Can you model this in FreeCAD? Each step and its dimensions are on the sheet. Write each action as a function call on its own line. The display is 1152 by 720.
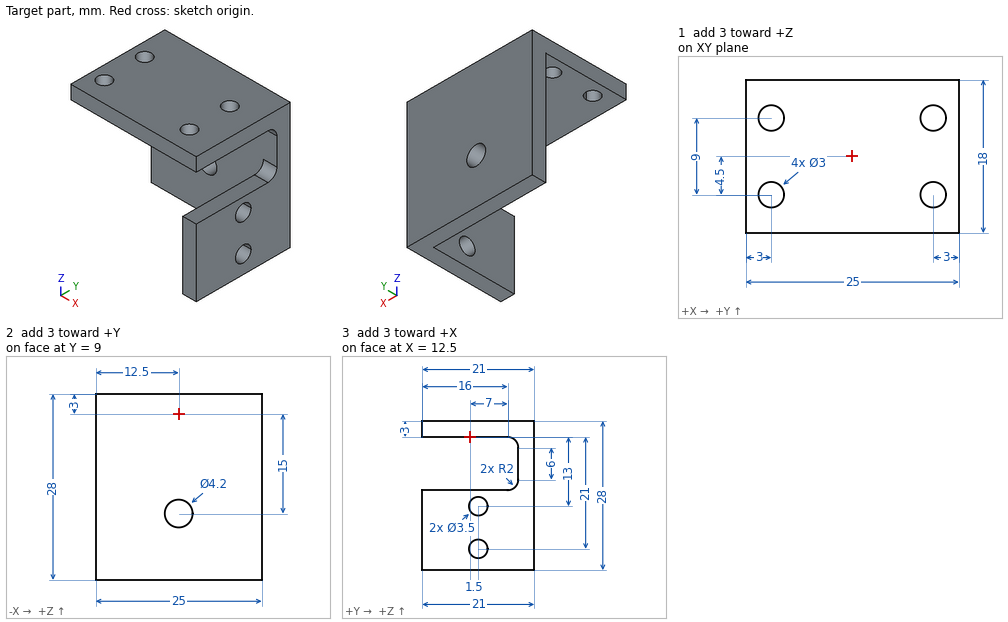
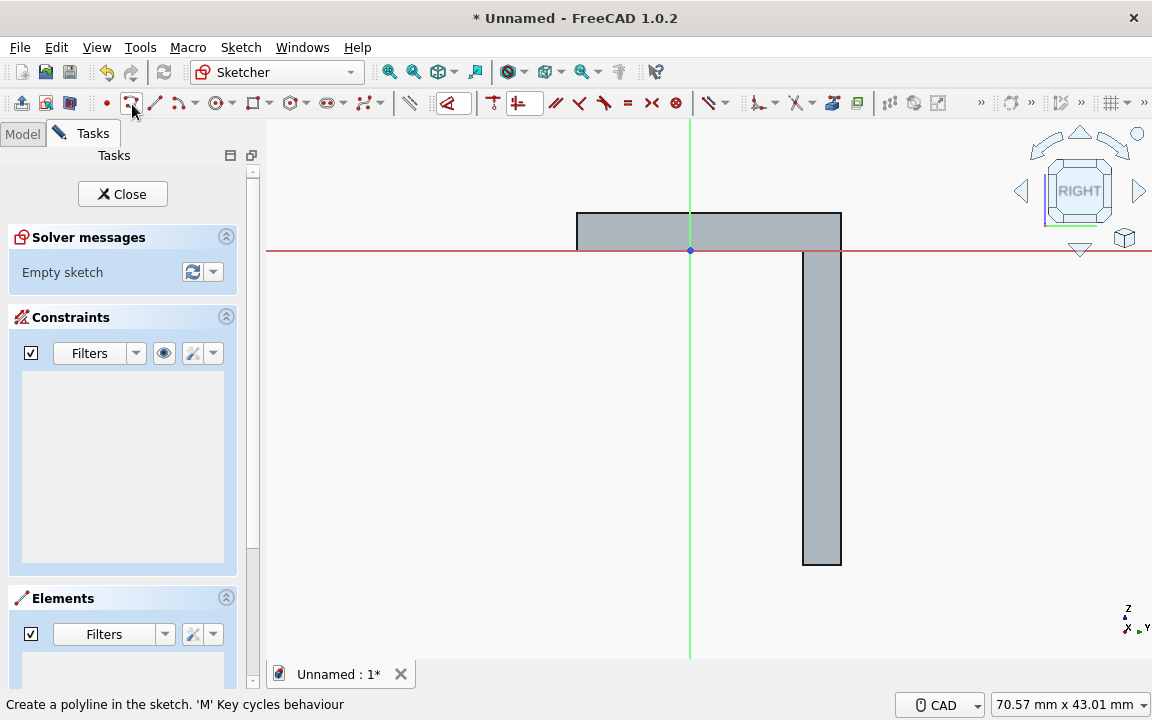
click(778, 251)
click(577, 260)
click(577, 213)
click(841, 213)
click(841, 565)
click(577, 565)
click(577, 376)
click(778, 376)
right_click(778, 376)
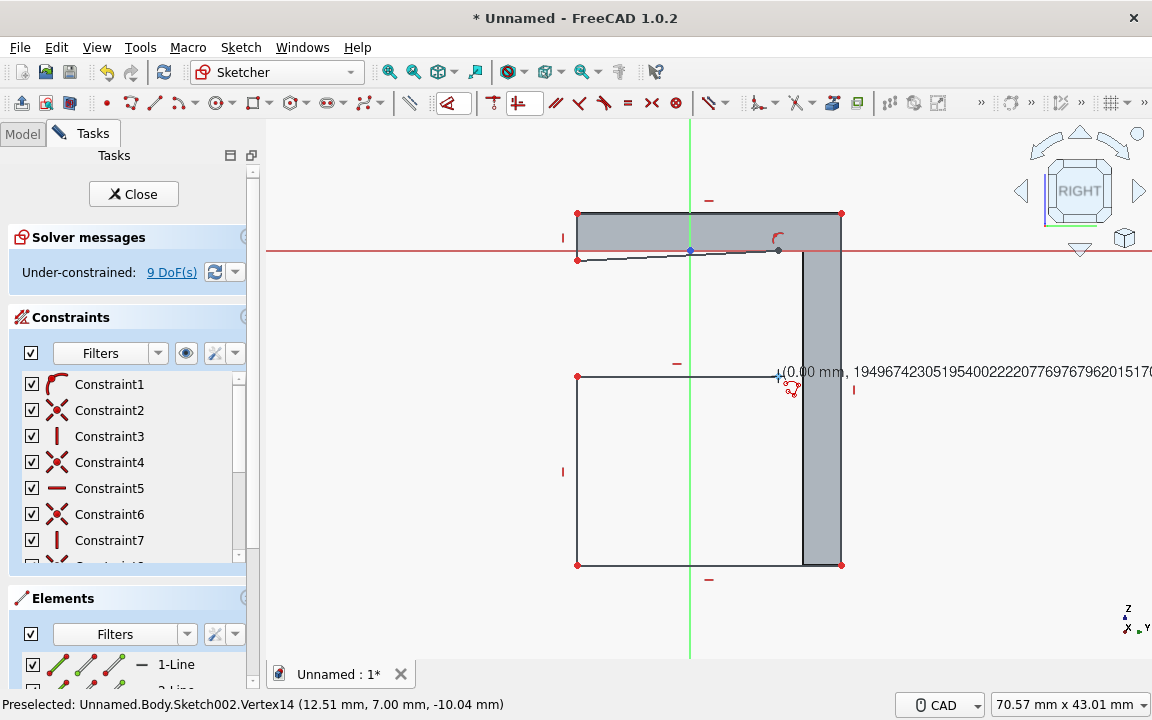
click(156, 104)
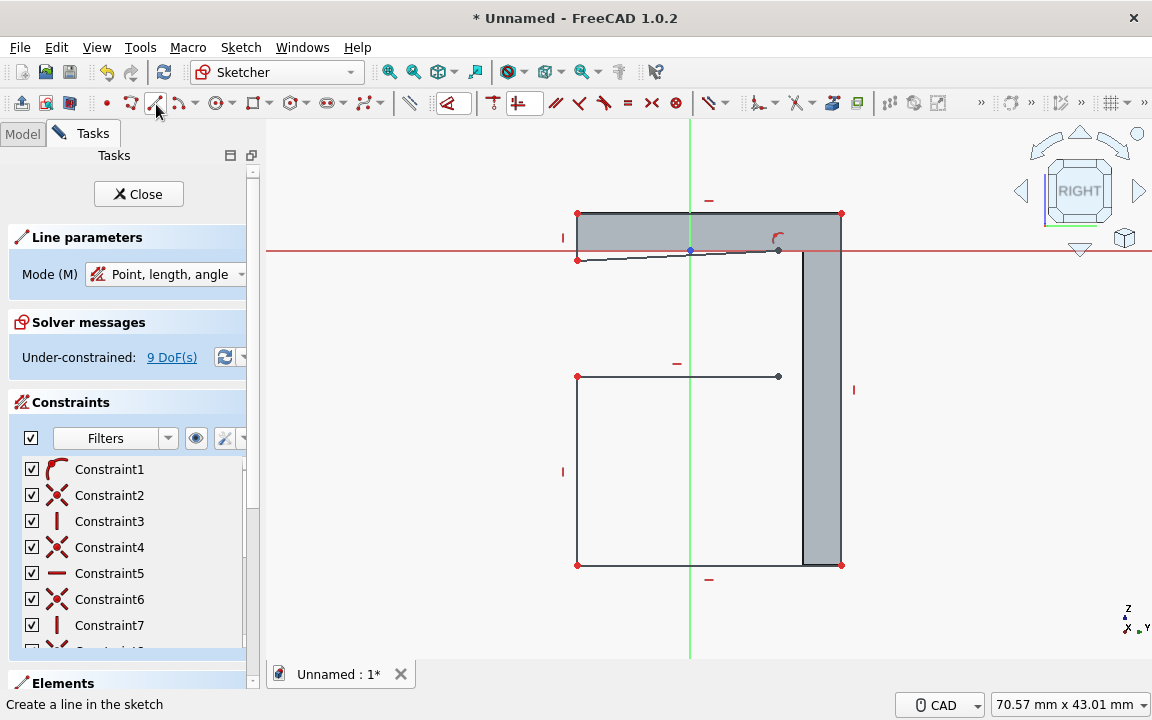
click(803, 351)
click(803, 276)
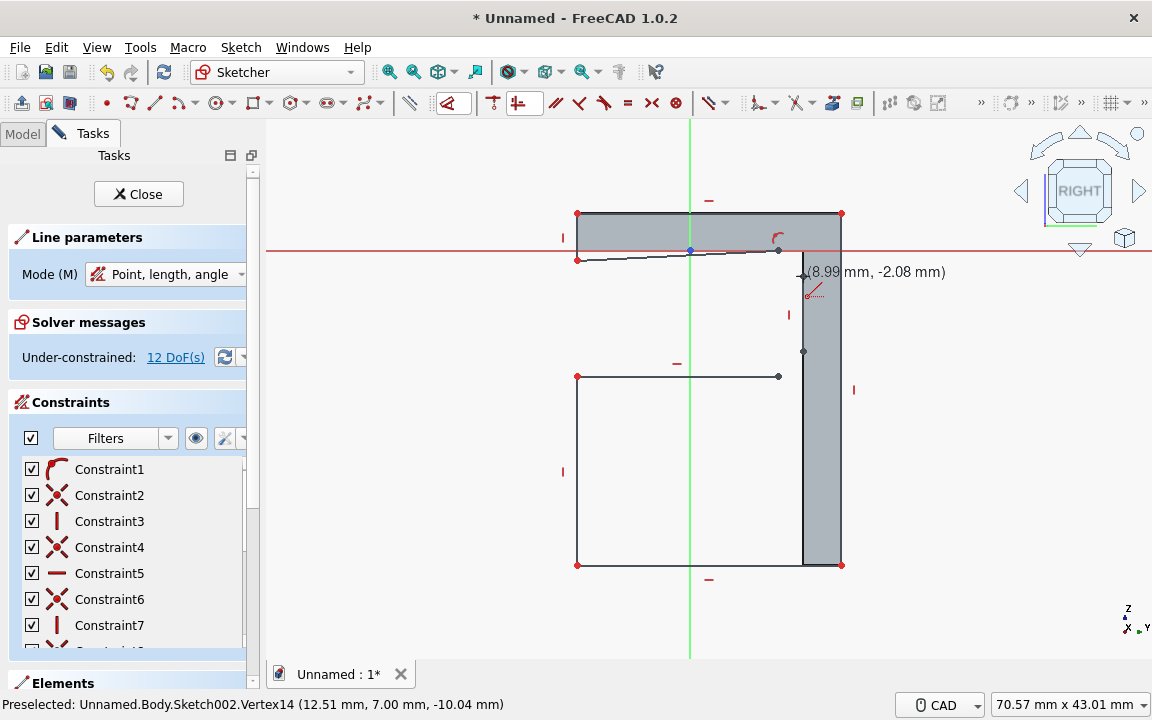
key(g)
key(3)
key(a)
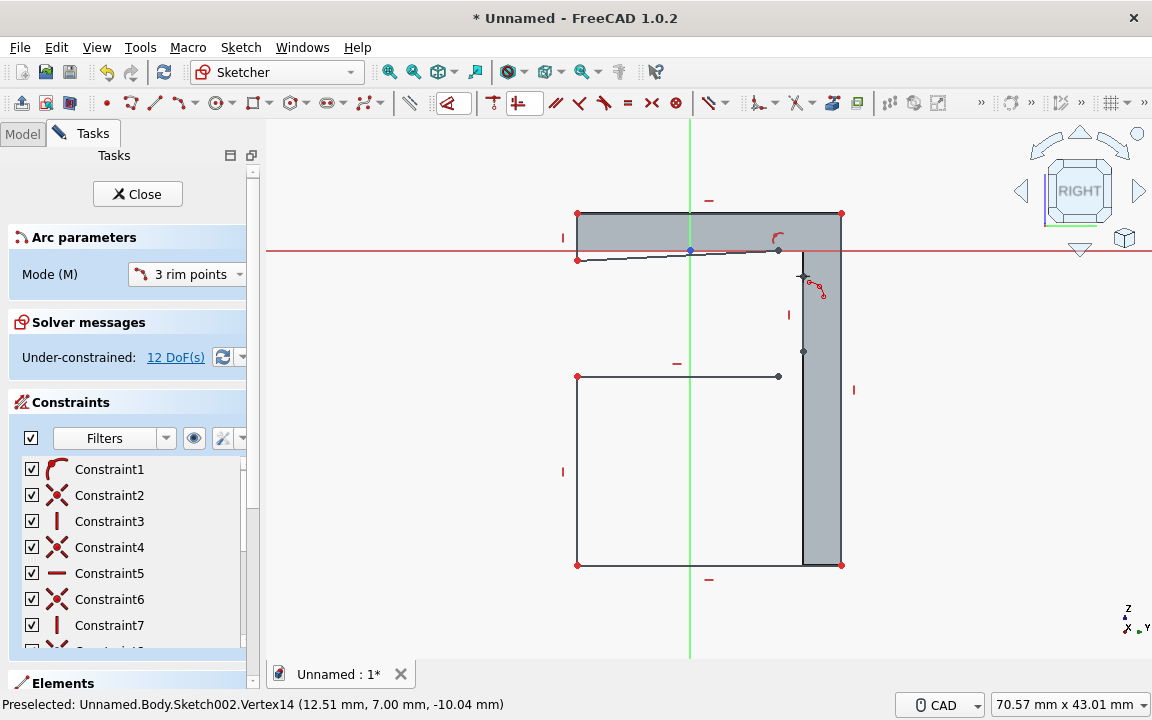
click(778, 377)
click(803, 352)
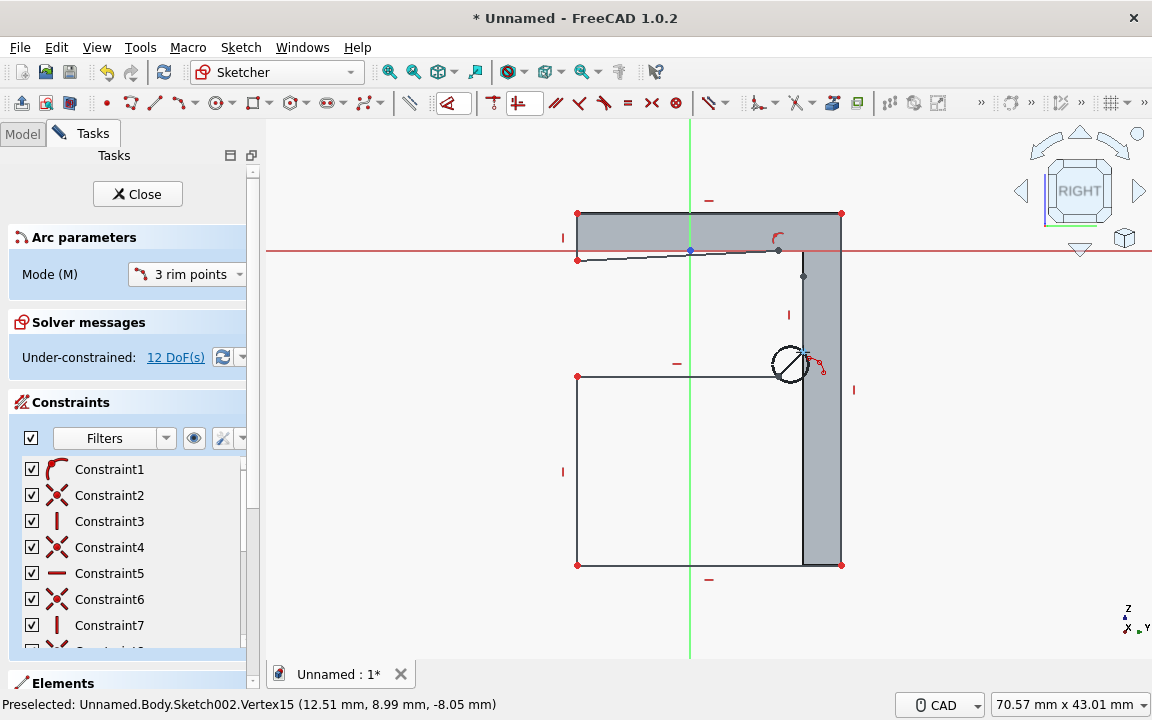
scroll(796, 369, up, 4)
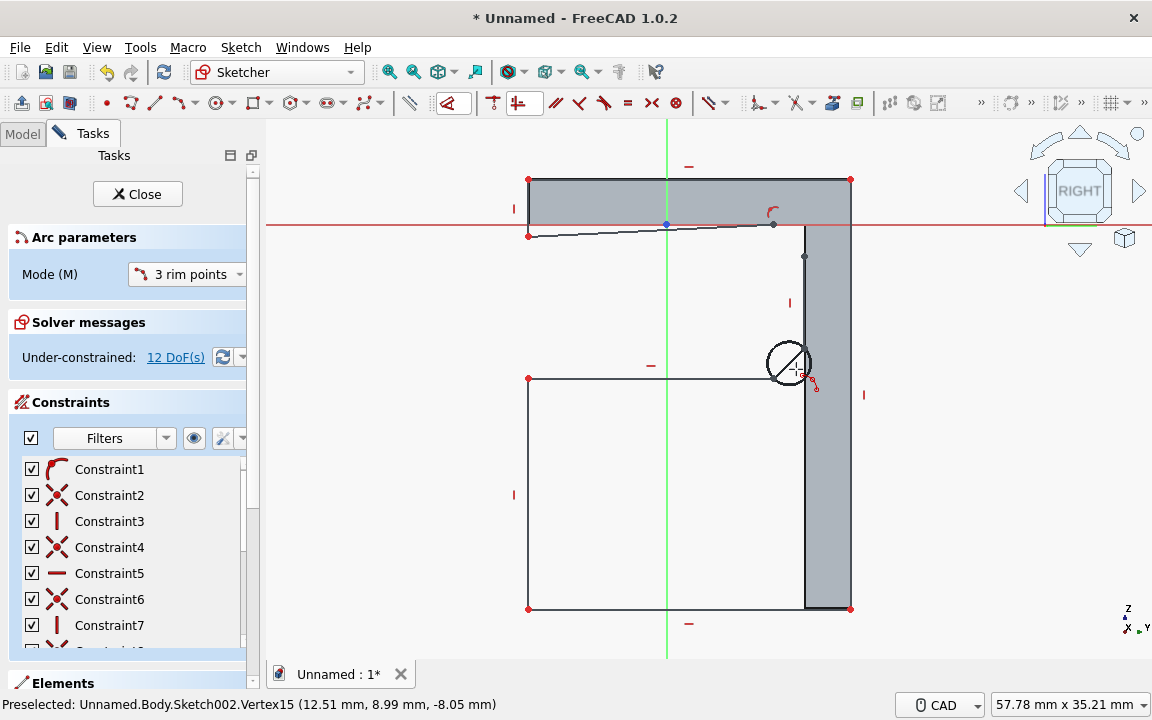
click(795, 369)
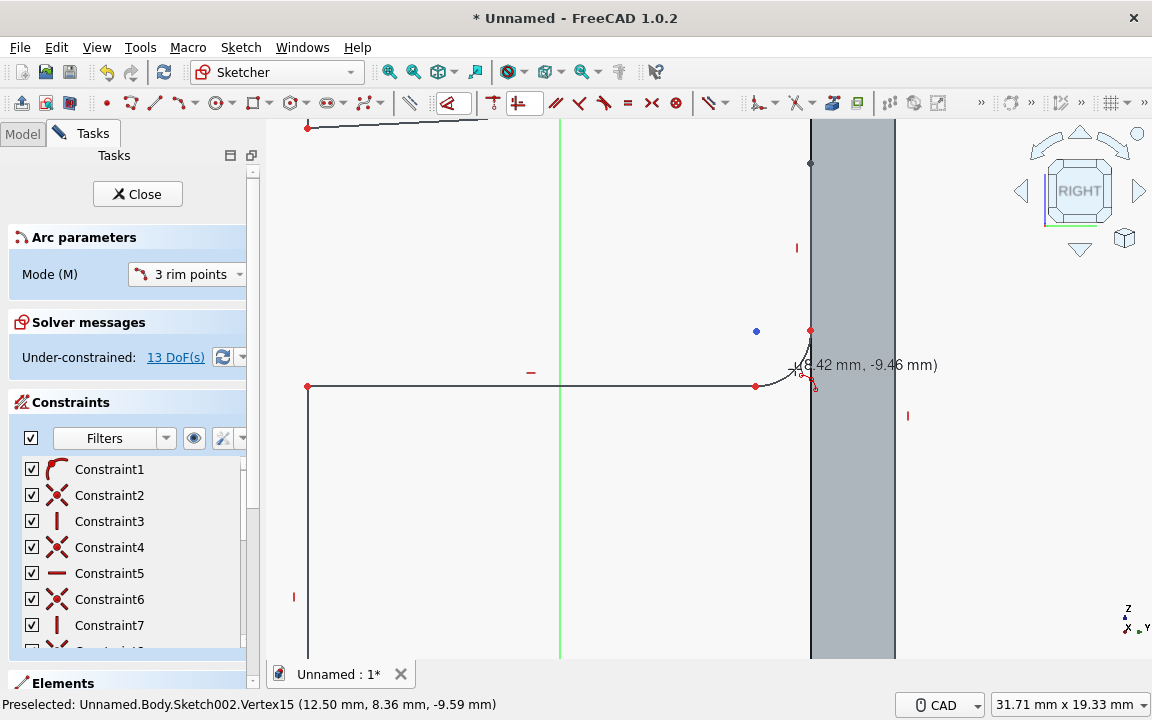
click(811, 164)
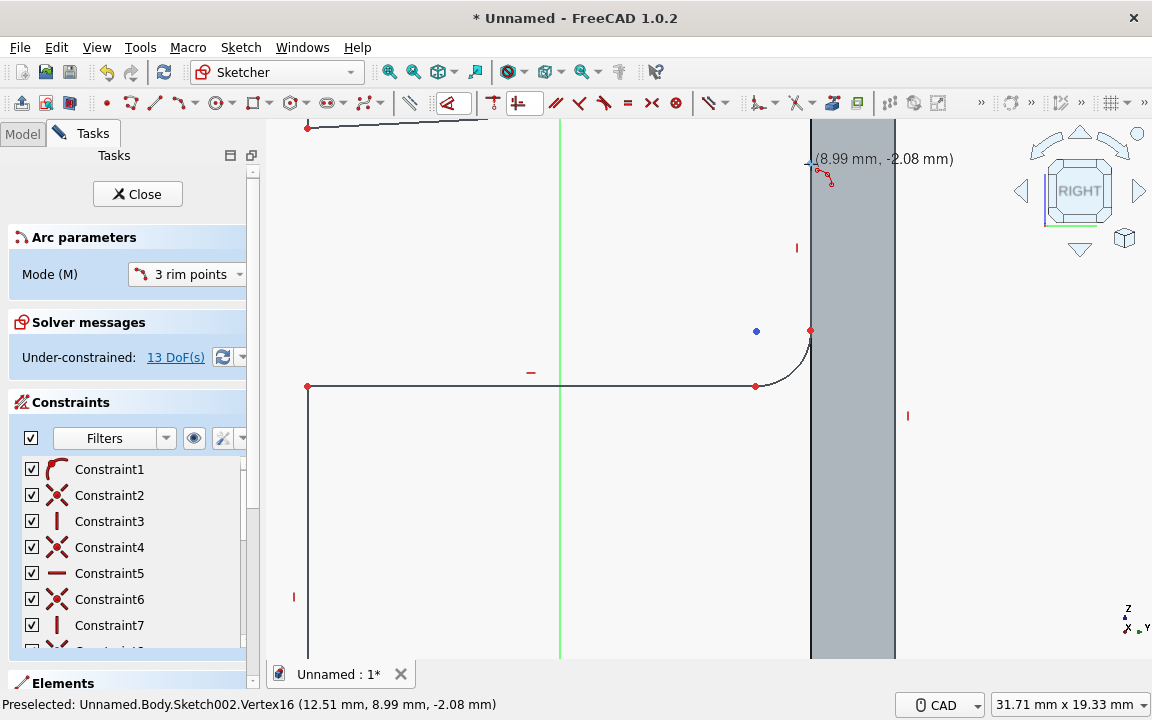
scroll(672, 369, down, 4)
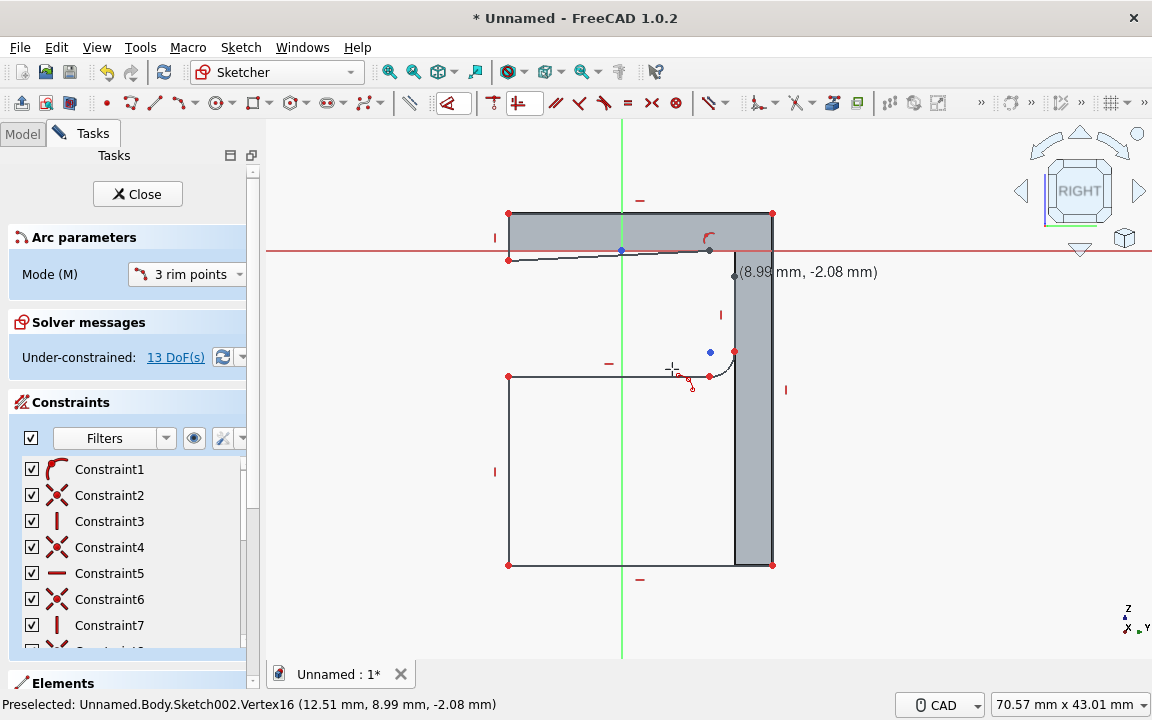
click(710, 251)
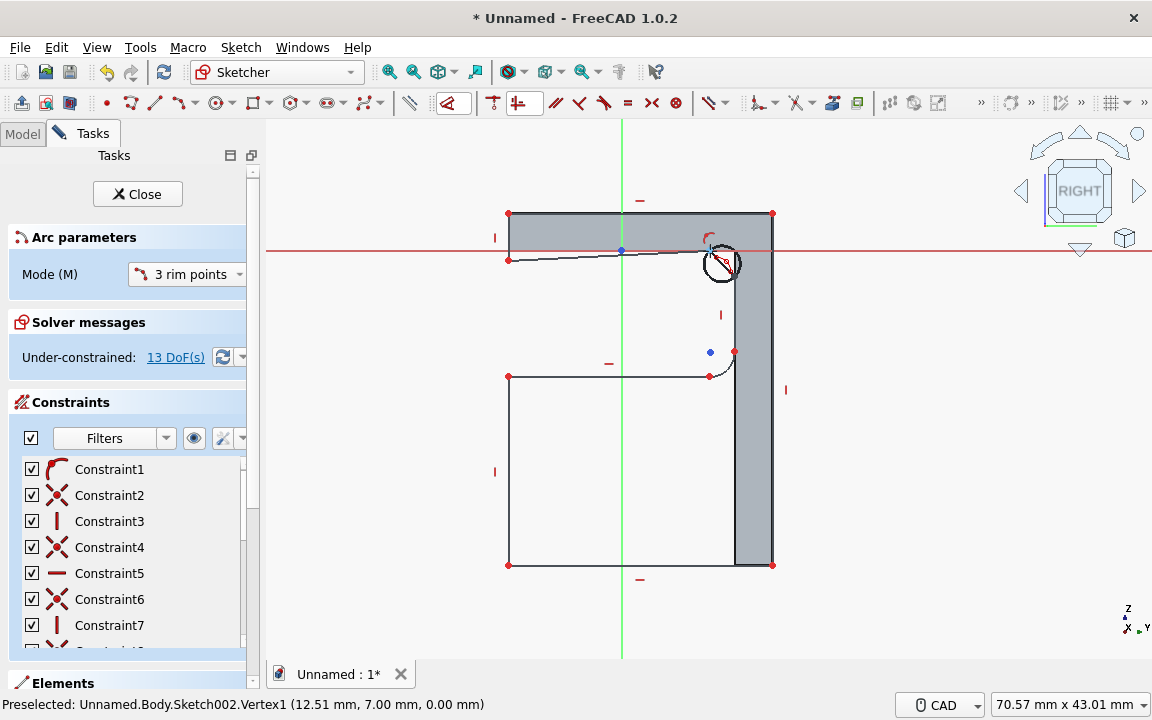
scroll(727, 258, up, 4)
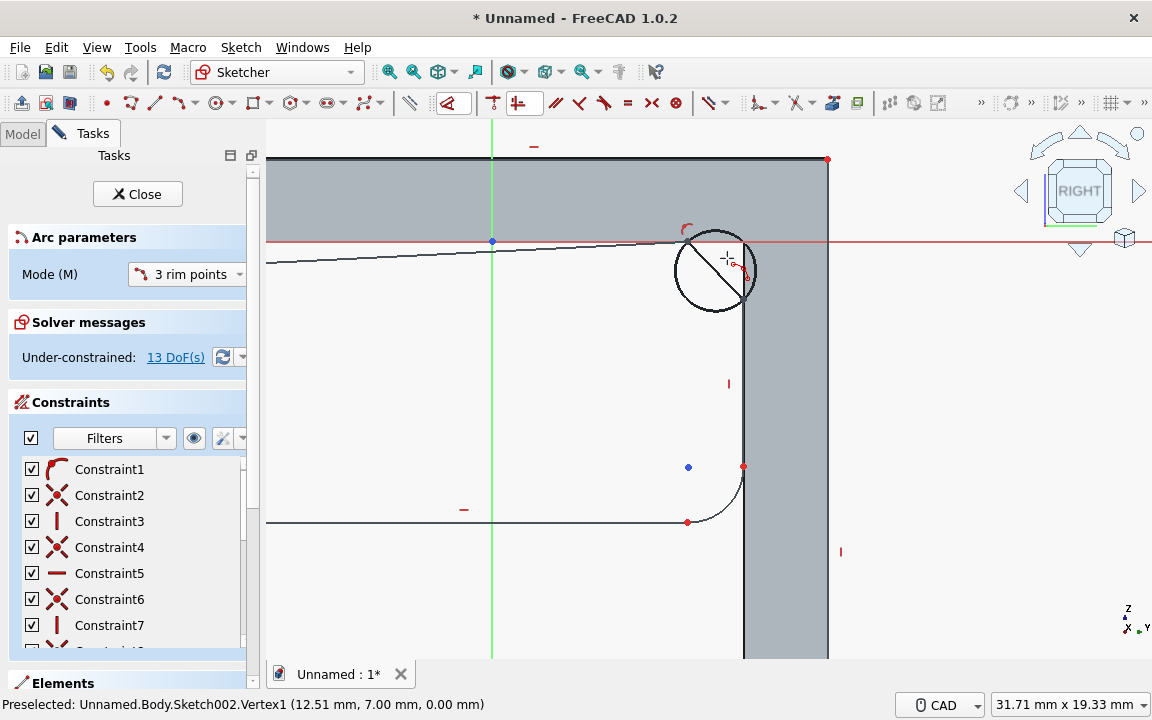
click(727, 258)